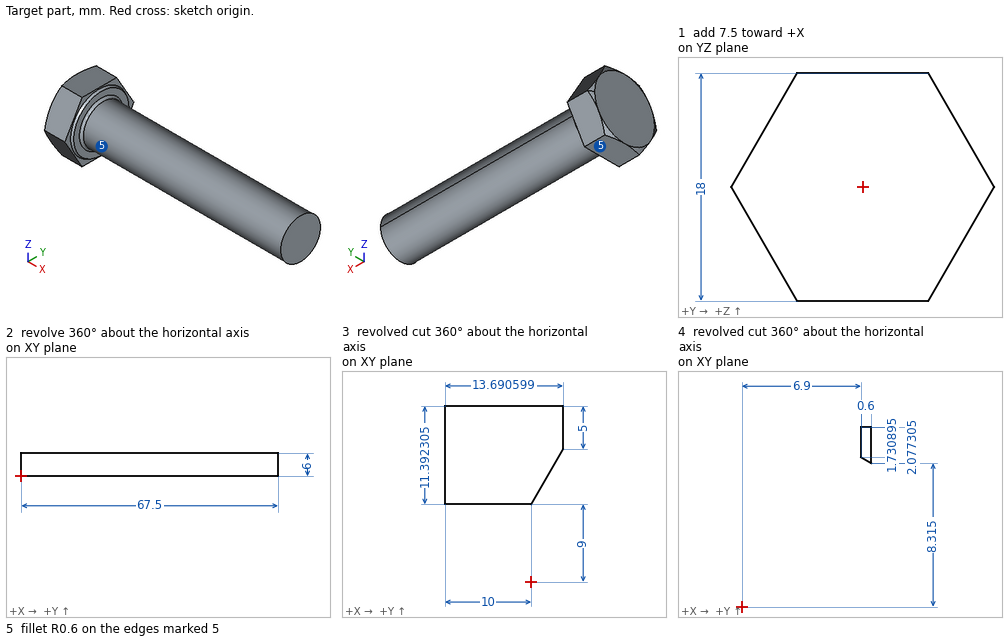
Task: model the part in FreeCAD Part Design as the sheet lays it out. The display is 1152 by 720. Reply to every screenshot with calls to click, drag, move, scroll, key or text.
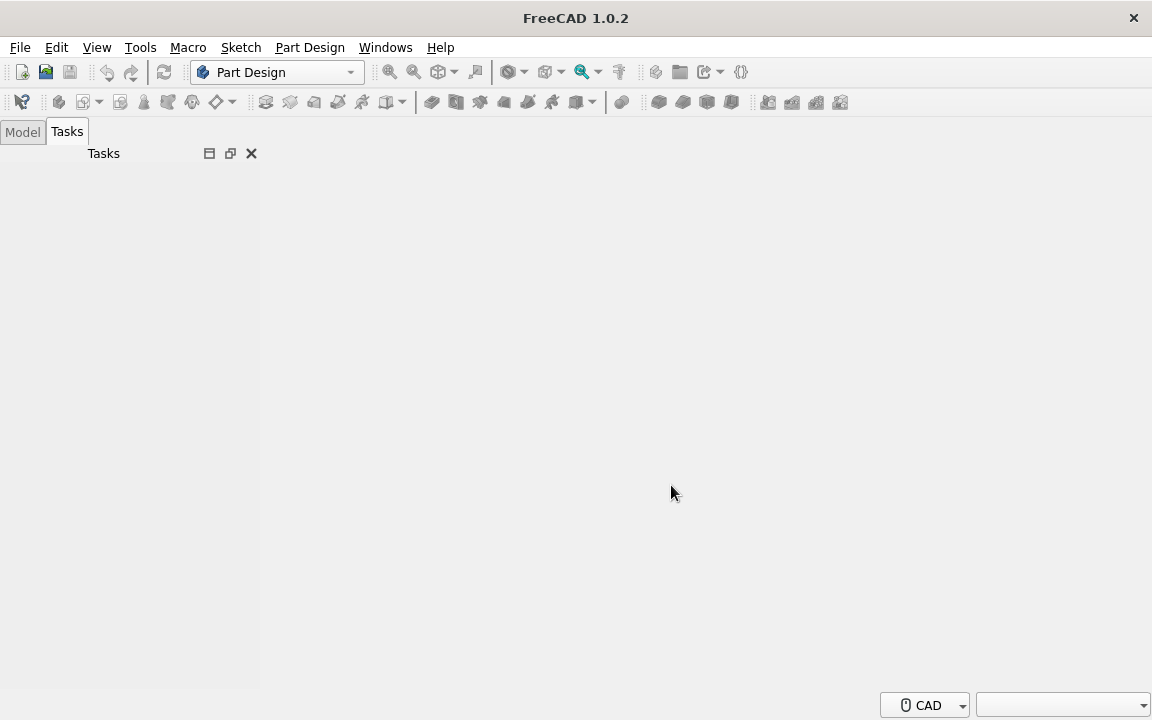
key(ctrl+n)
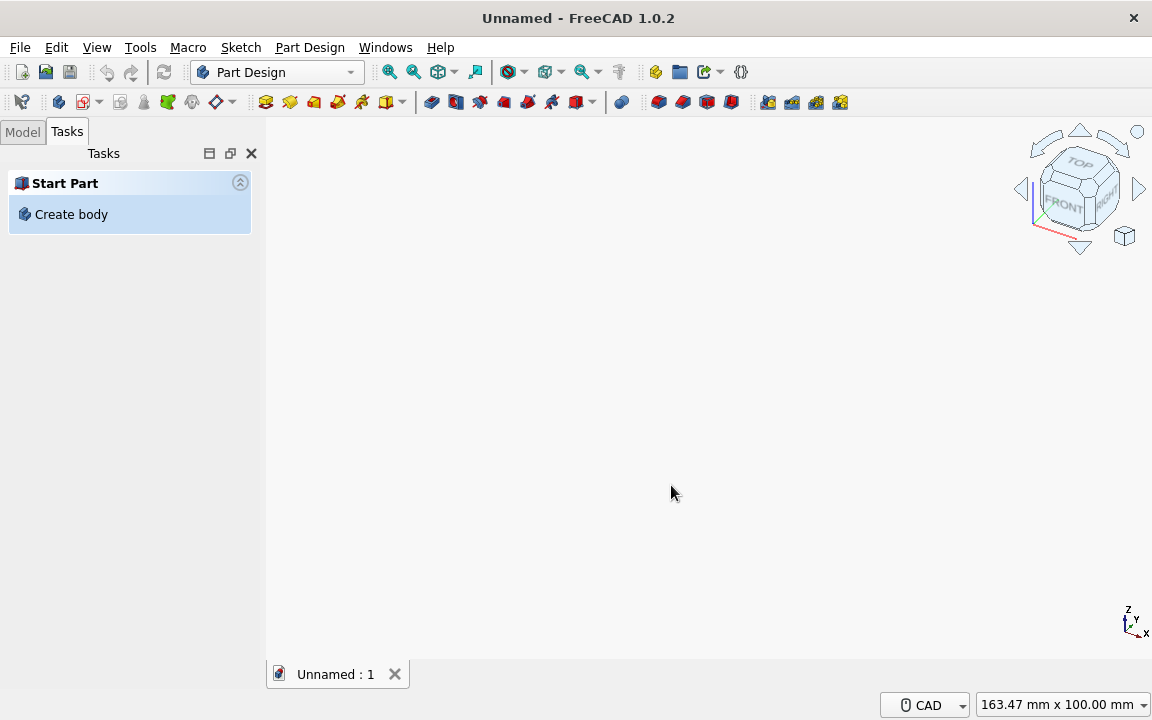
click(84, 102)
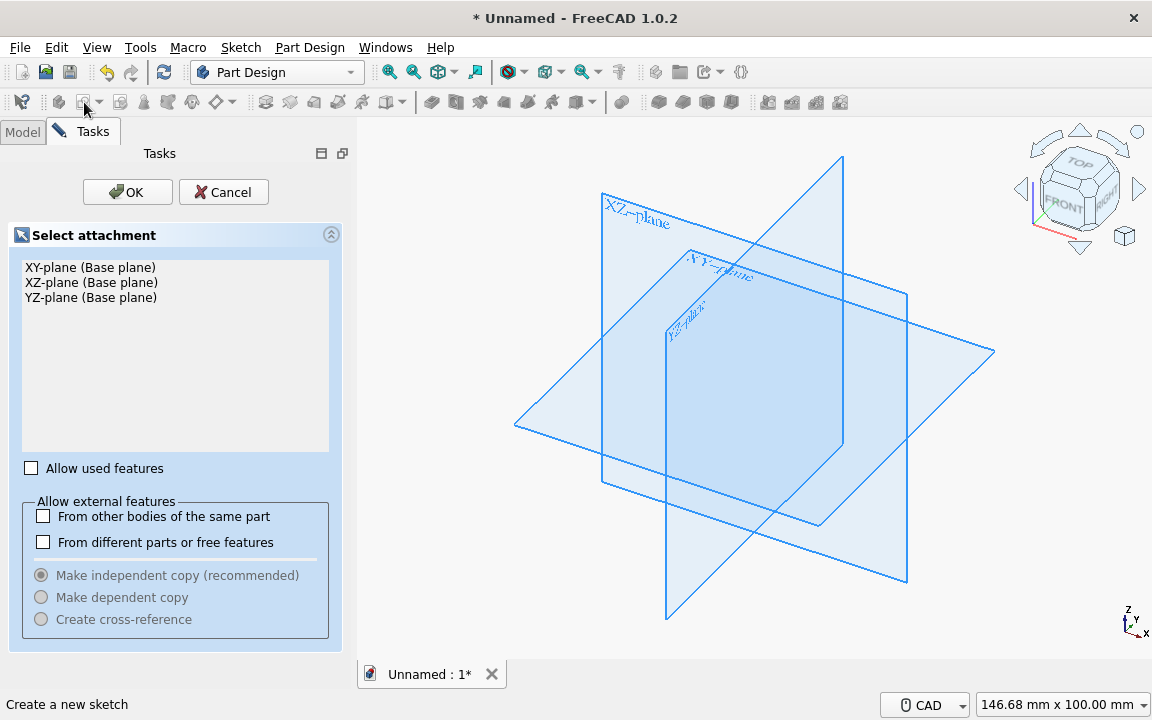
click(82, 298)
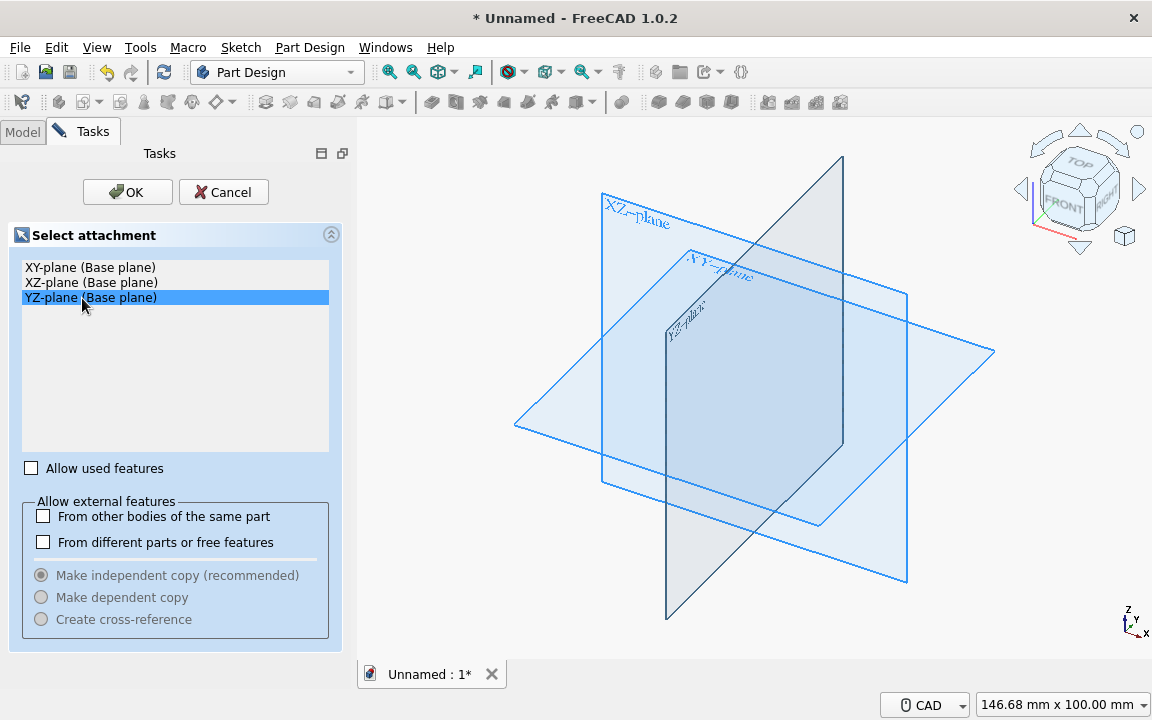
click(128, 192)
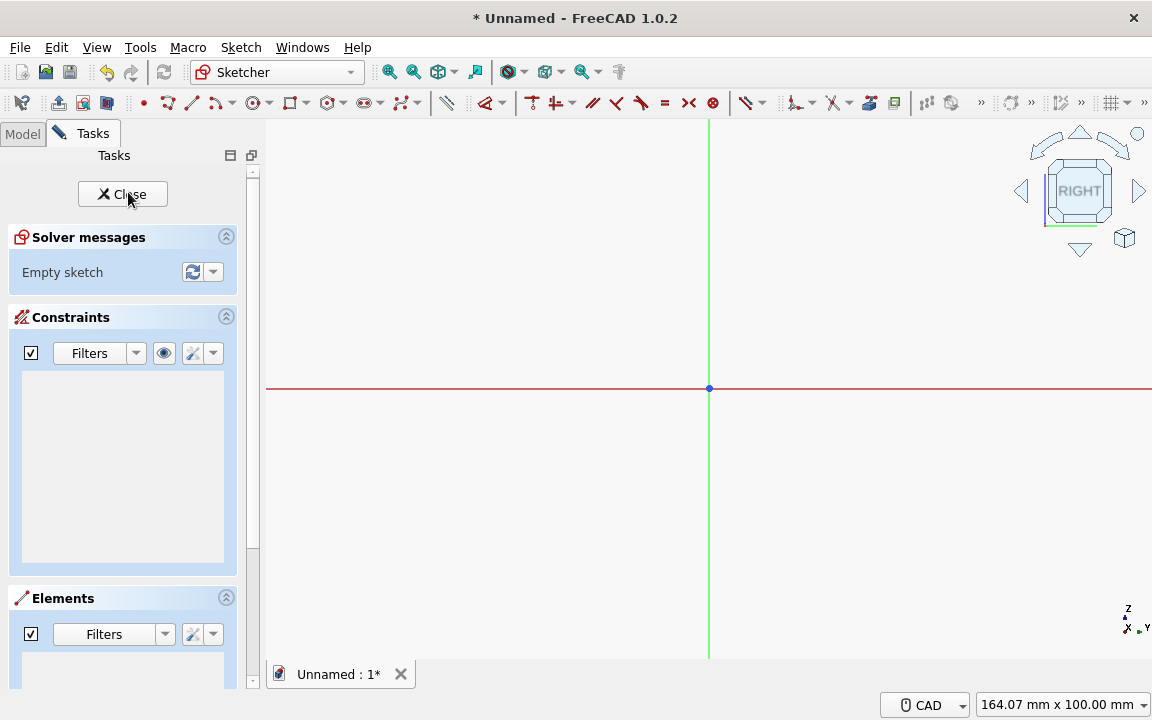
scroll(739, 389, up, 6)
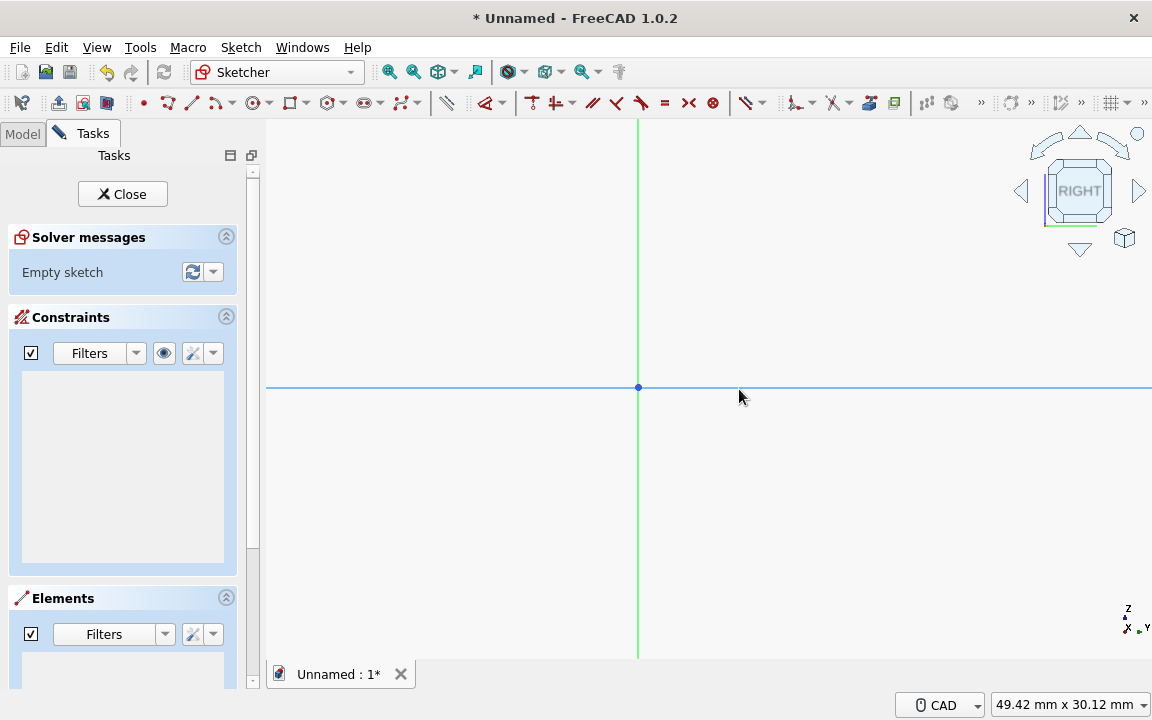
click(328, 104)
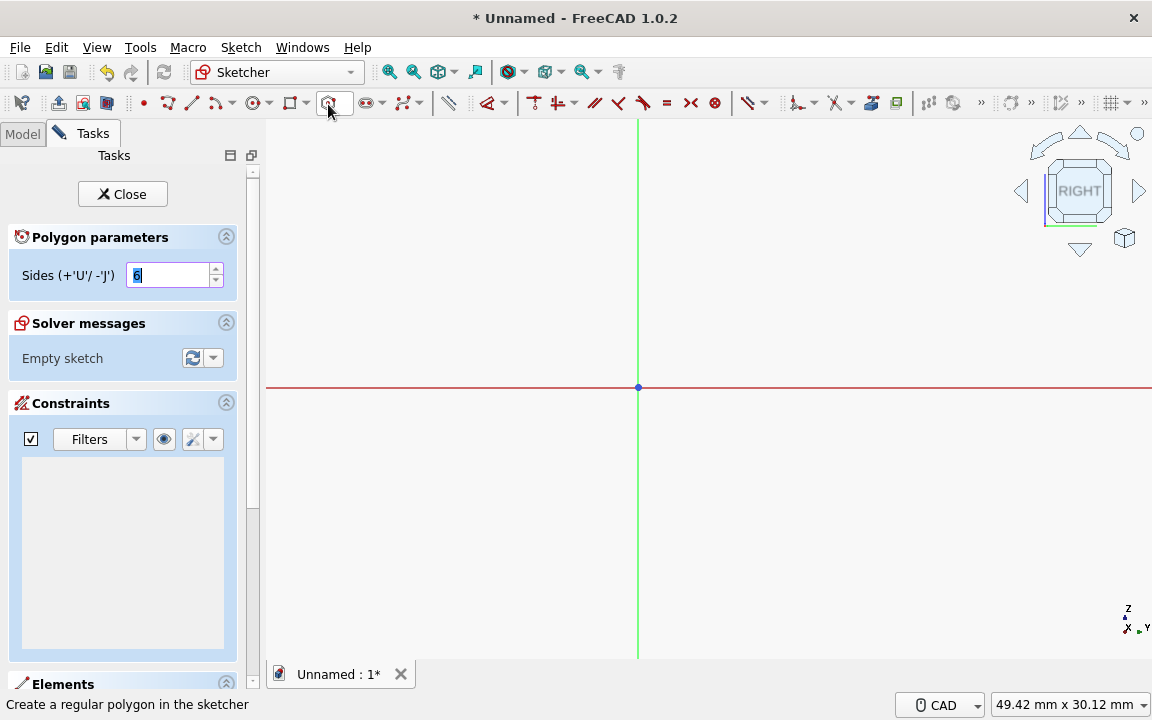
click(638, 388)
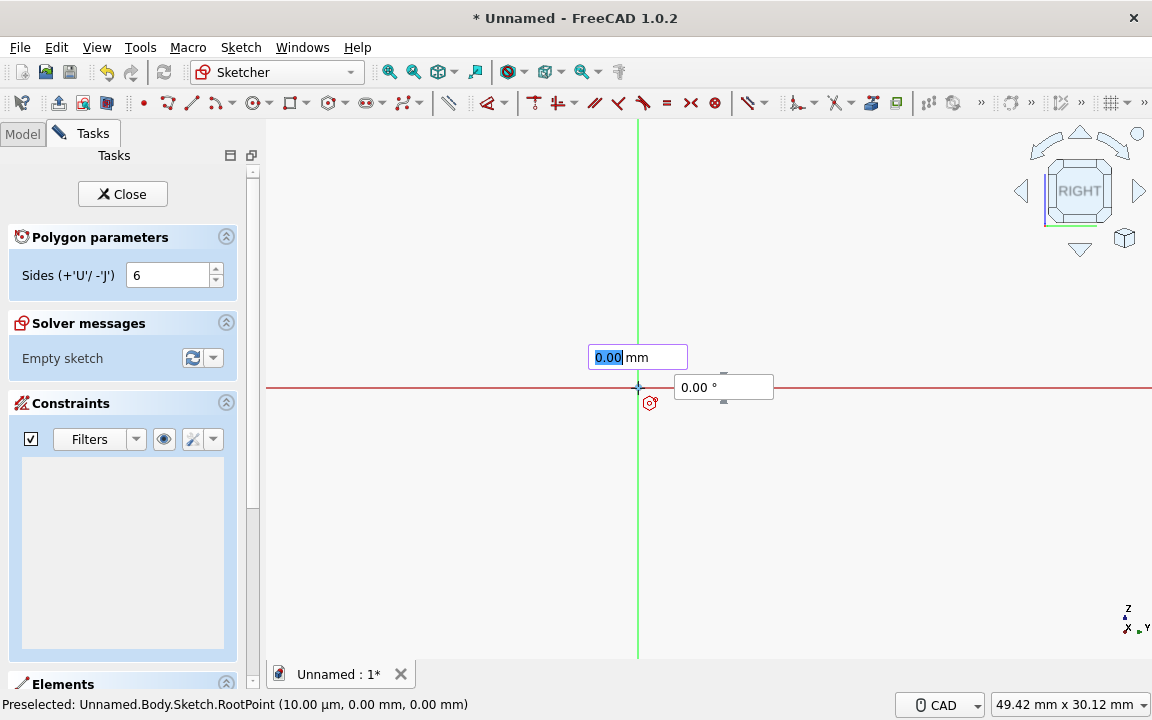
click(824, 388)
right_click(824, 388)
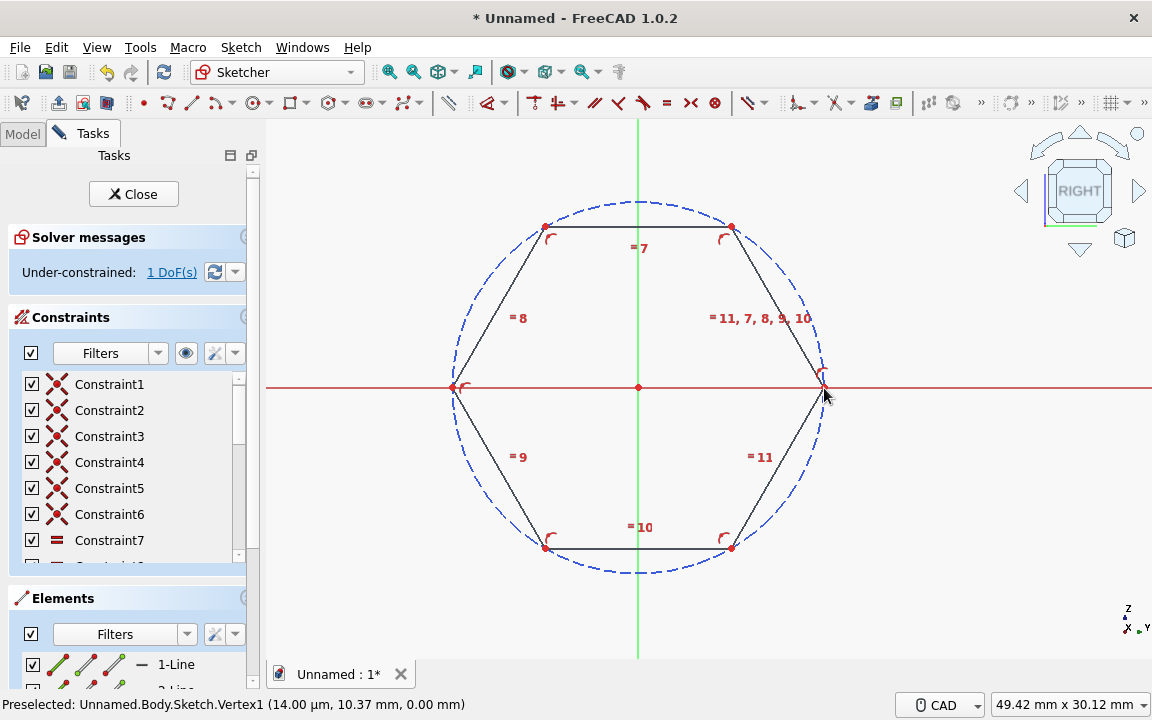
click(488, 104)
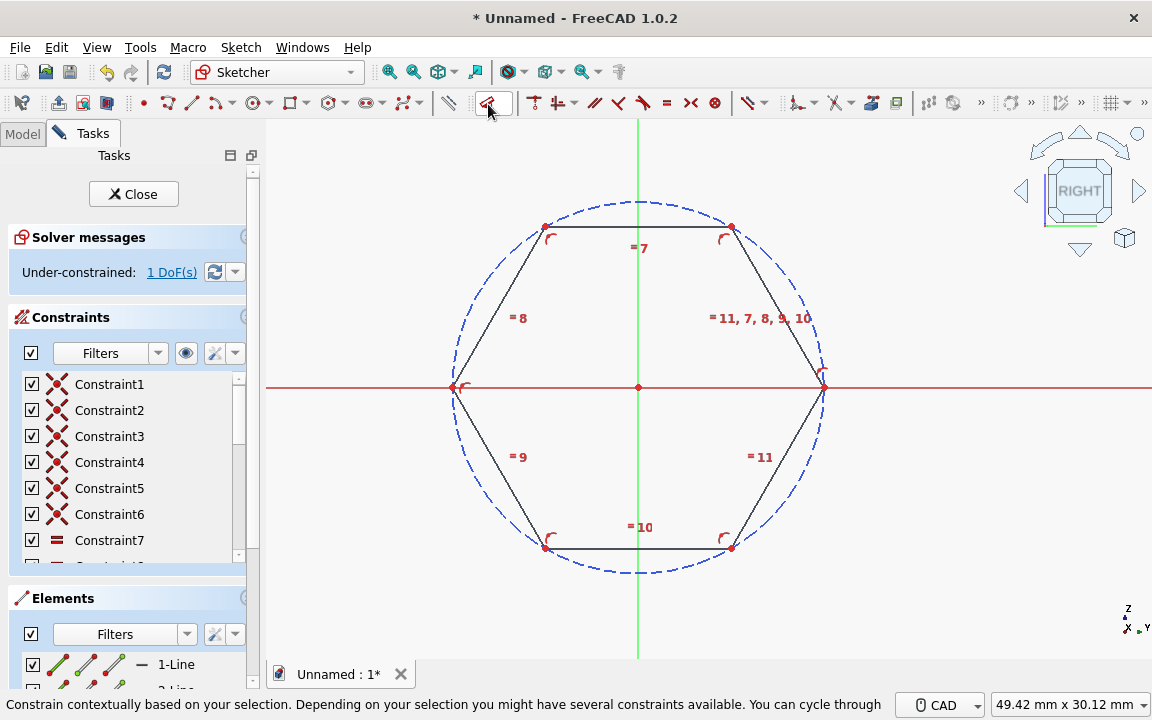
click(545, 549)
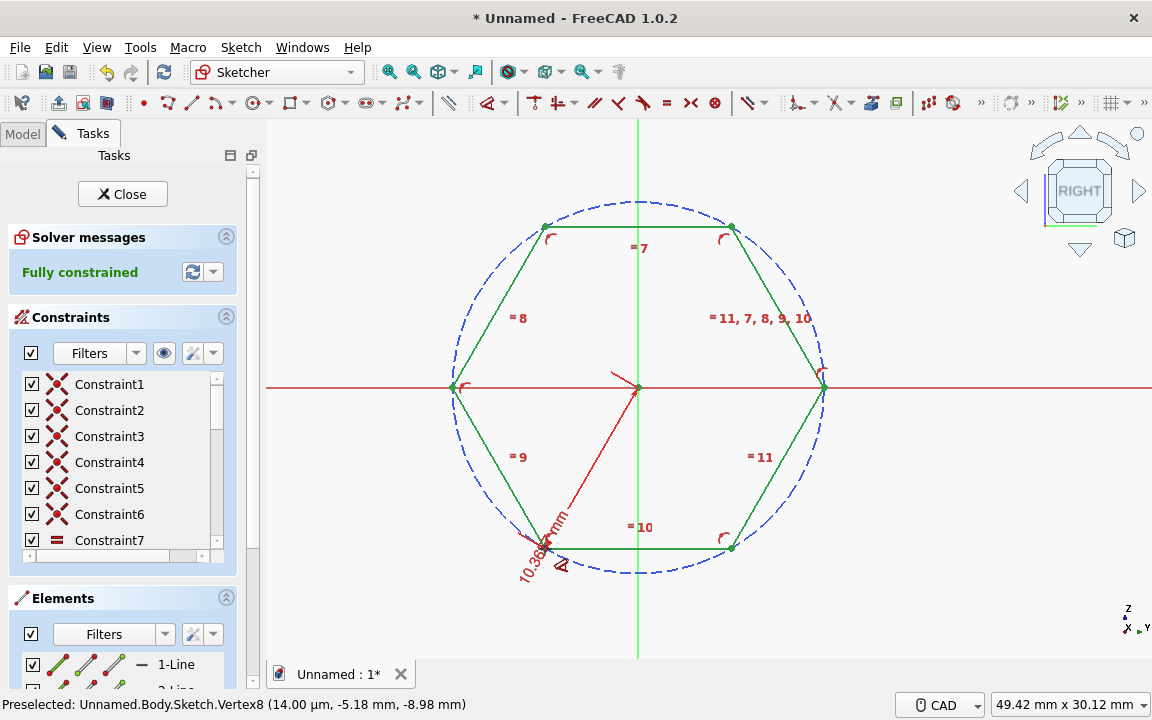
click(731, 227)
click(765, 314)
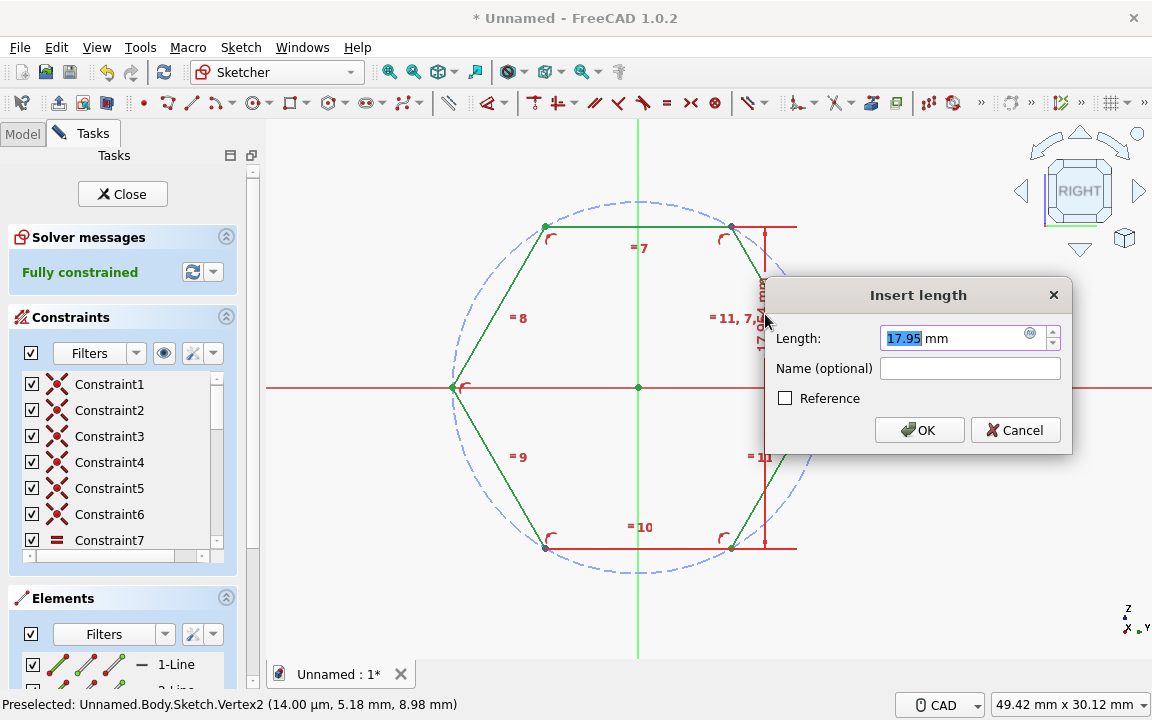
text(18)
key(Return)
key(Escape)